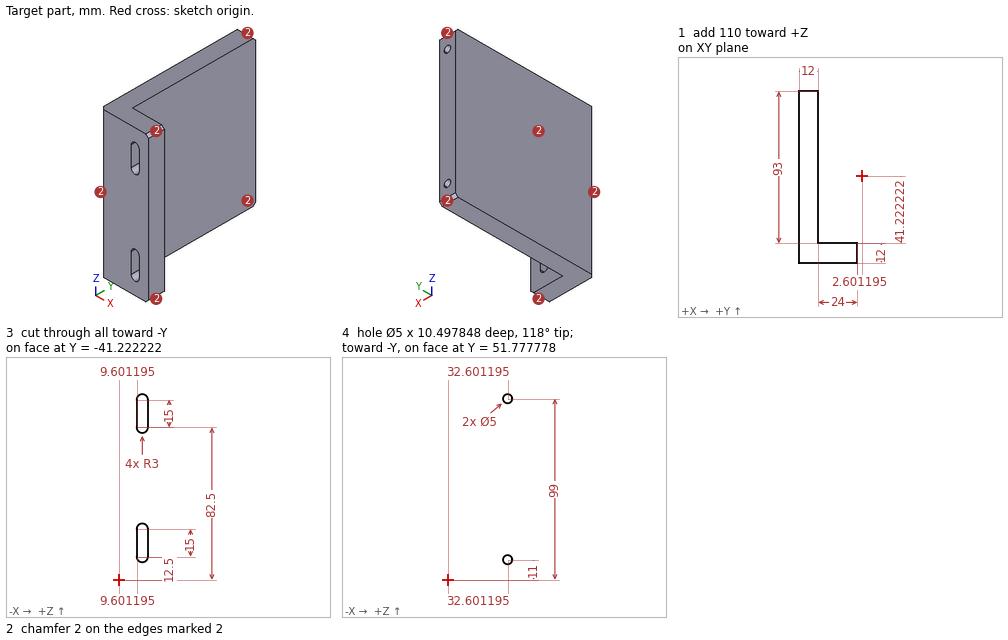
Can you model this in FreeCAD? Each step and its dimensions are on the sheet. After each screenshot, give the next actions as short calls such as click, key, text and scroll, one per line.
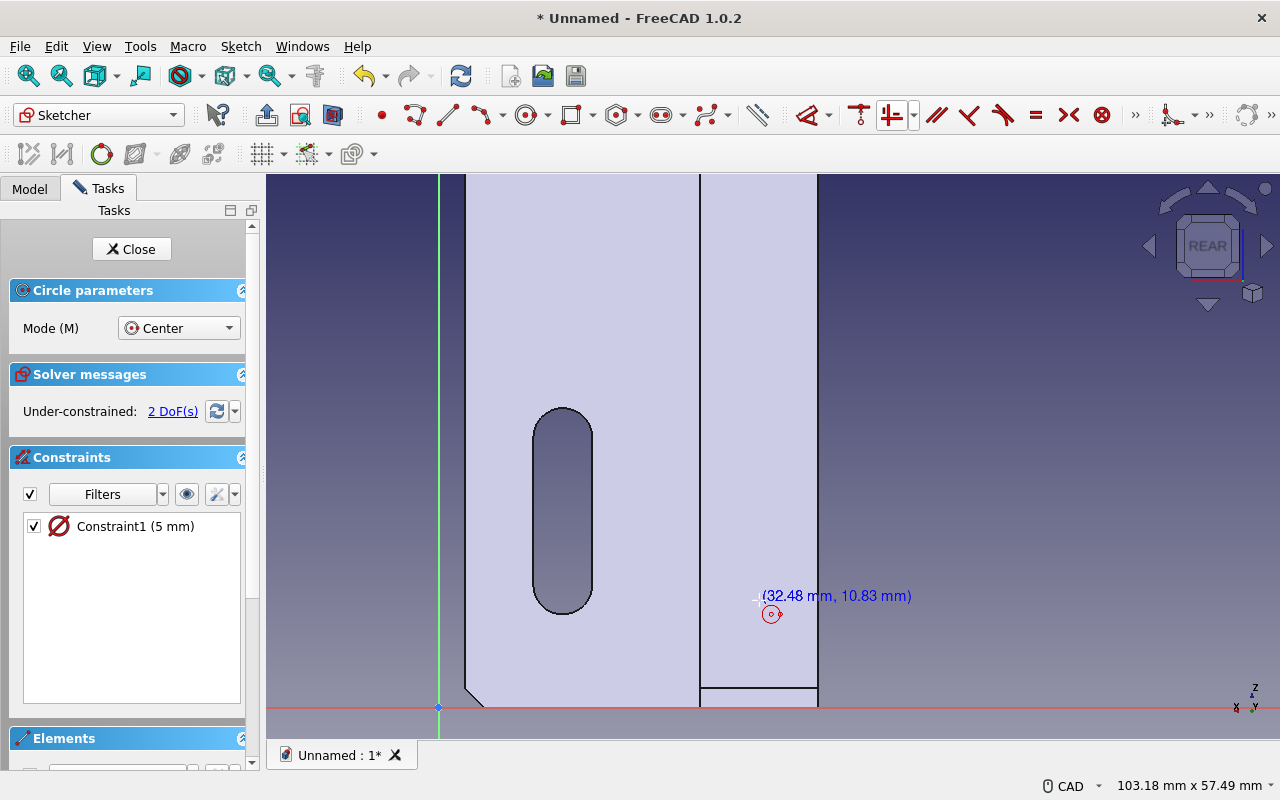
click(759, 600)
move(777, 582)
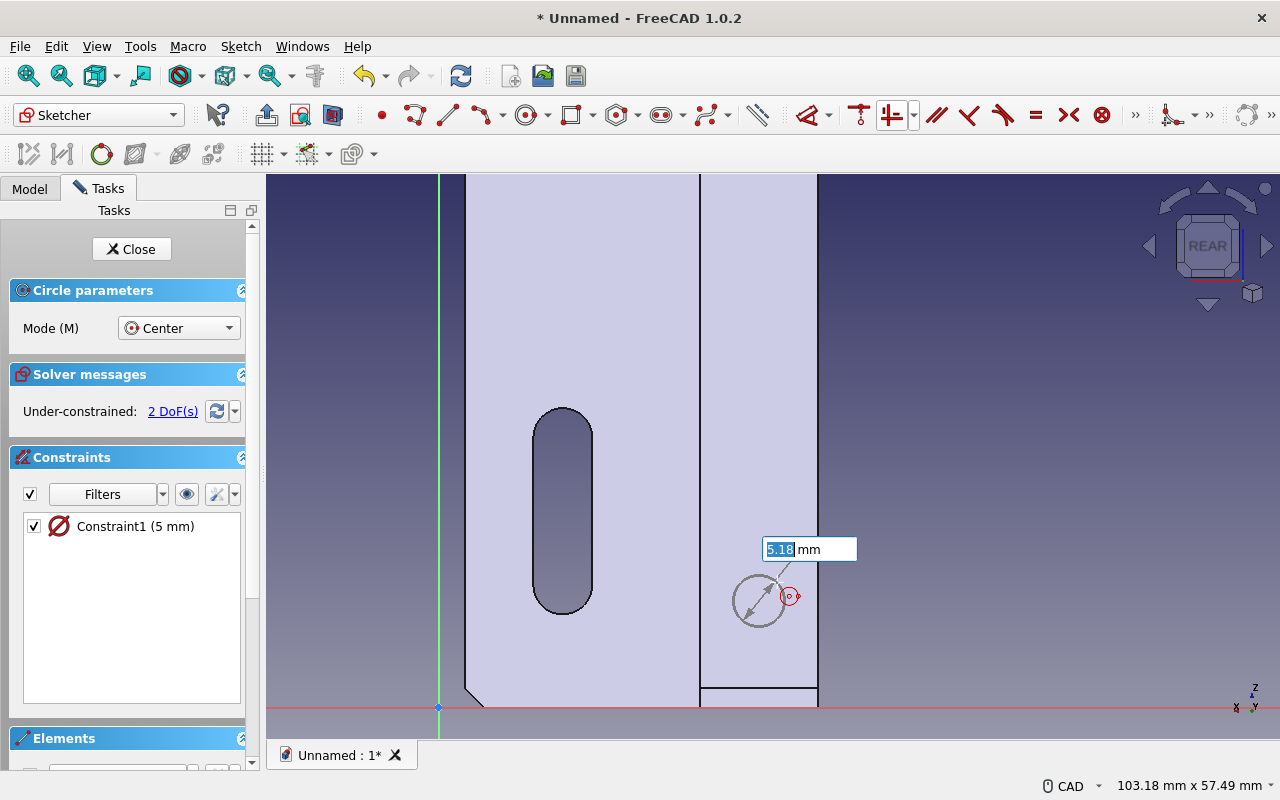
text(5)
key(Return)
key(Escape)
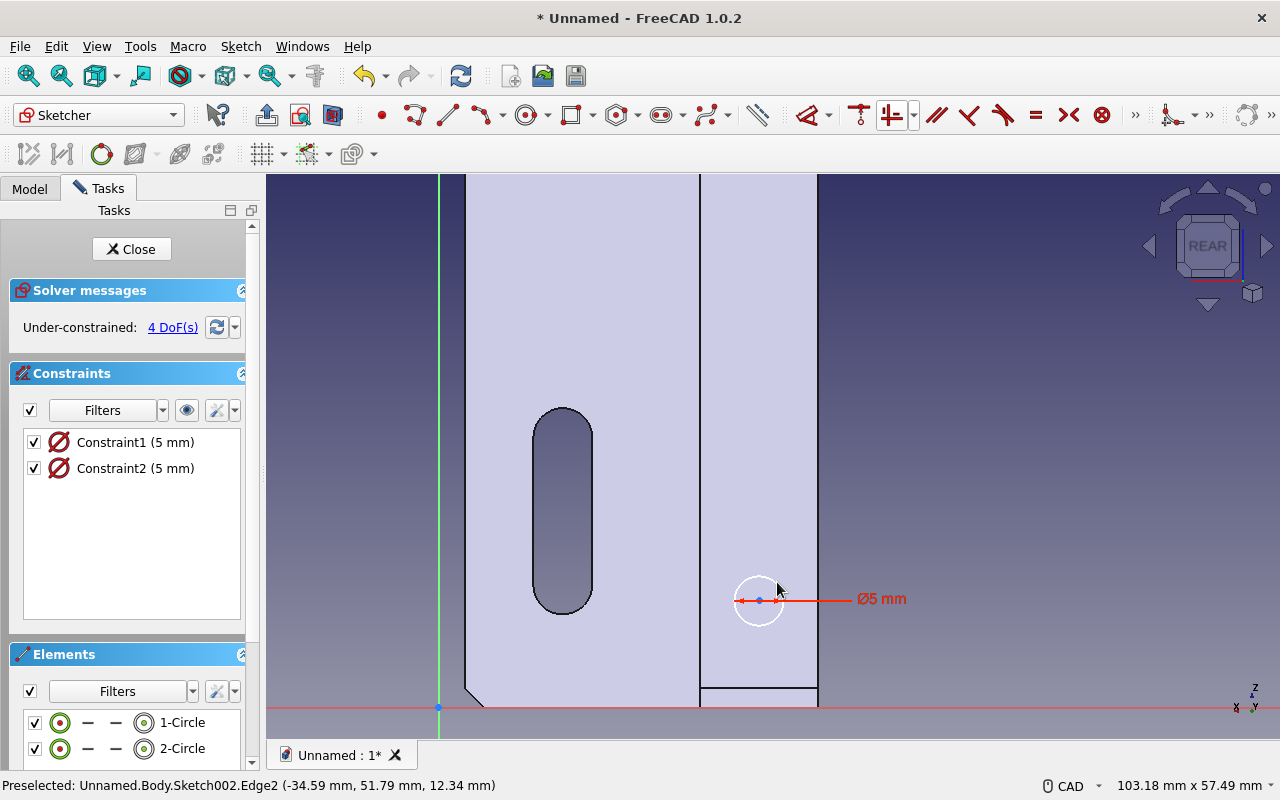
click(806, 116)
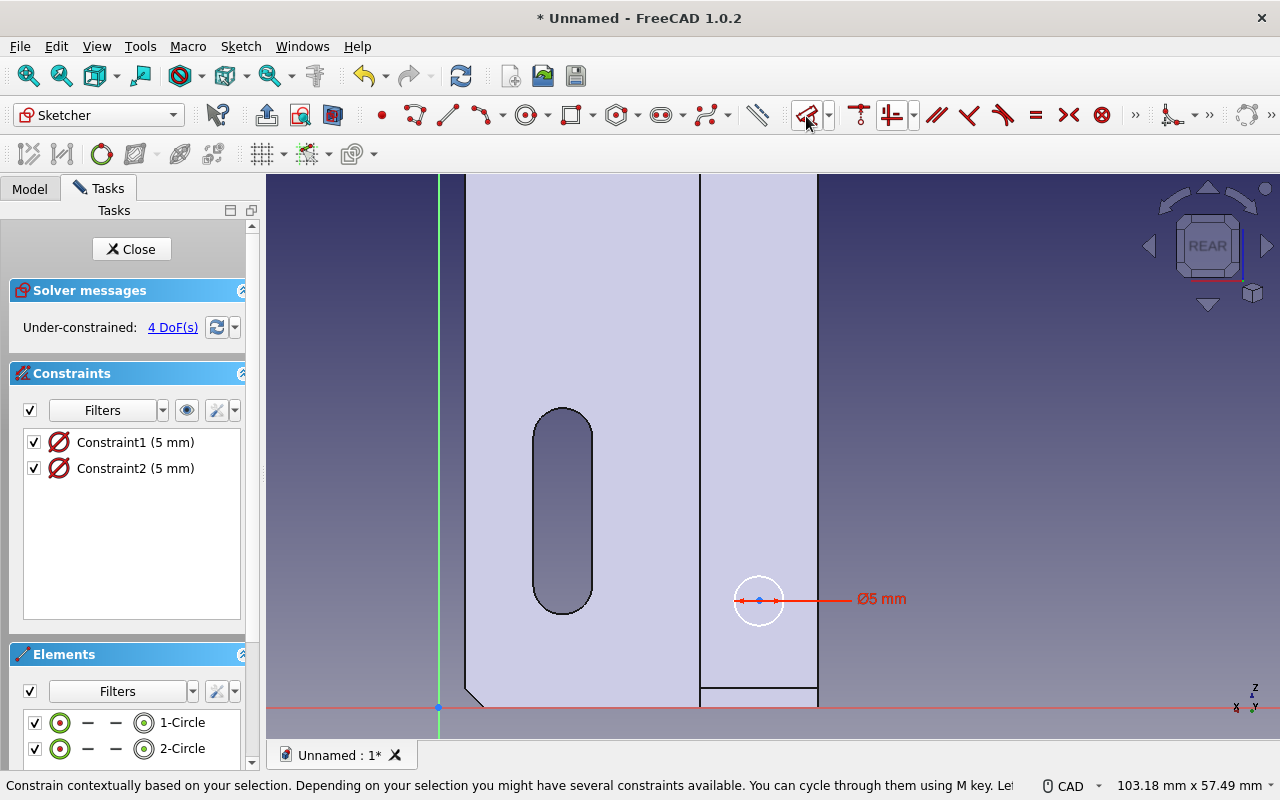
scroll(759, 600, down, 5)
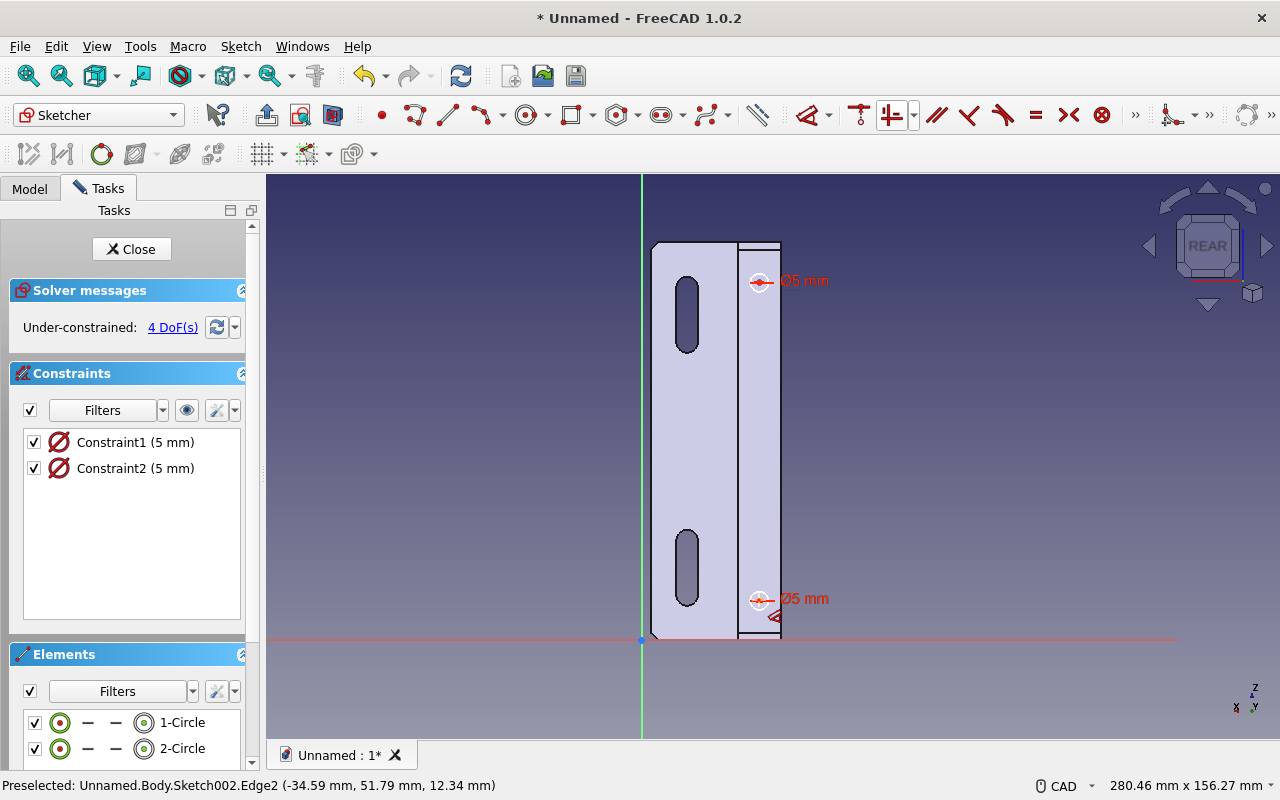
click(759, 283)
click(608, 461)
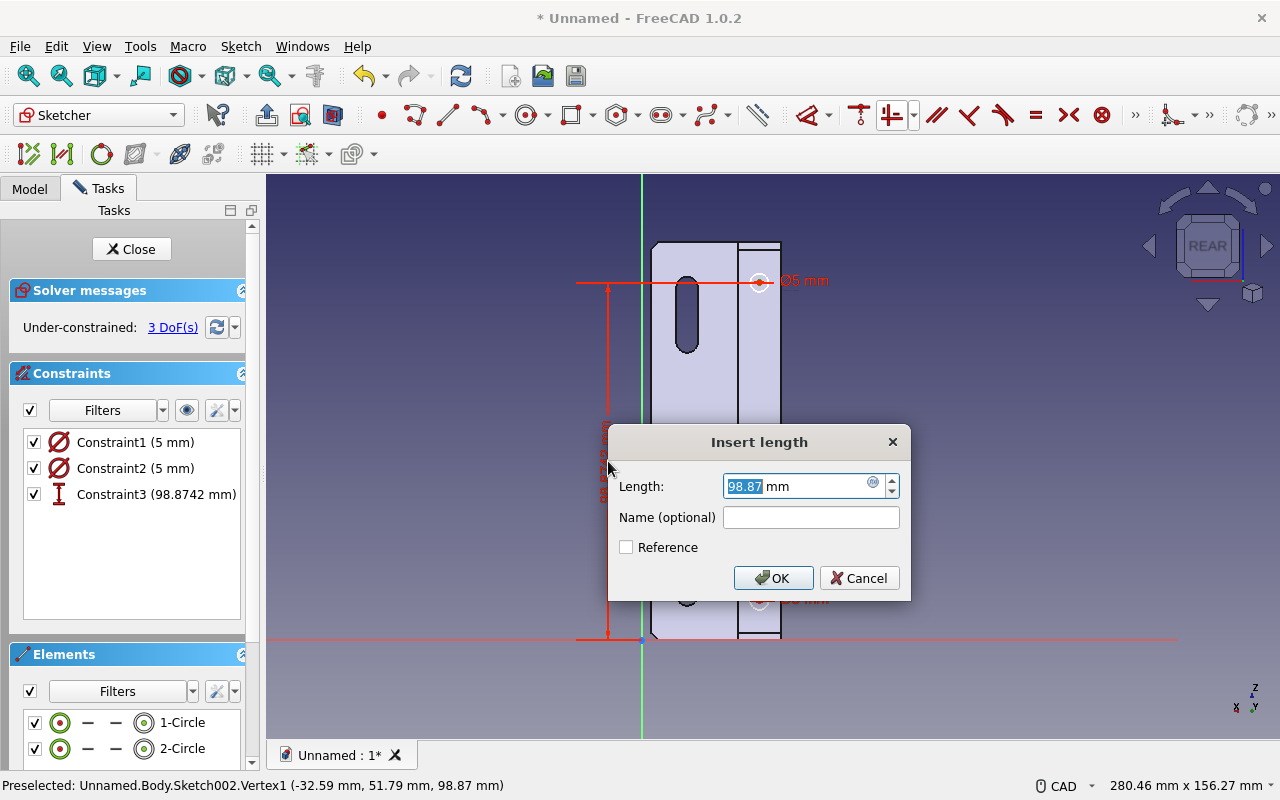
text(99)
key(Return)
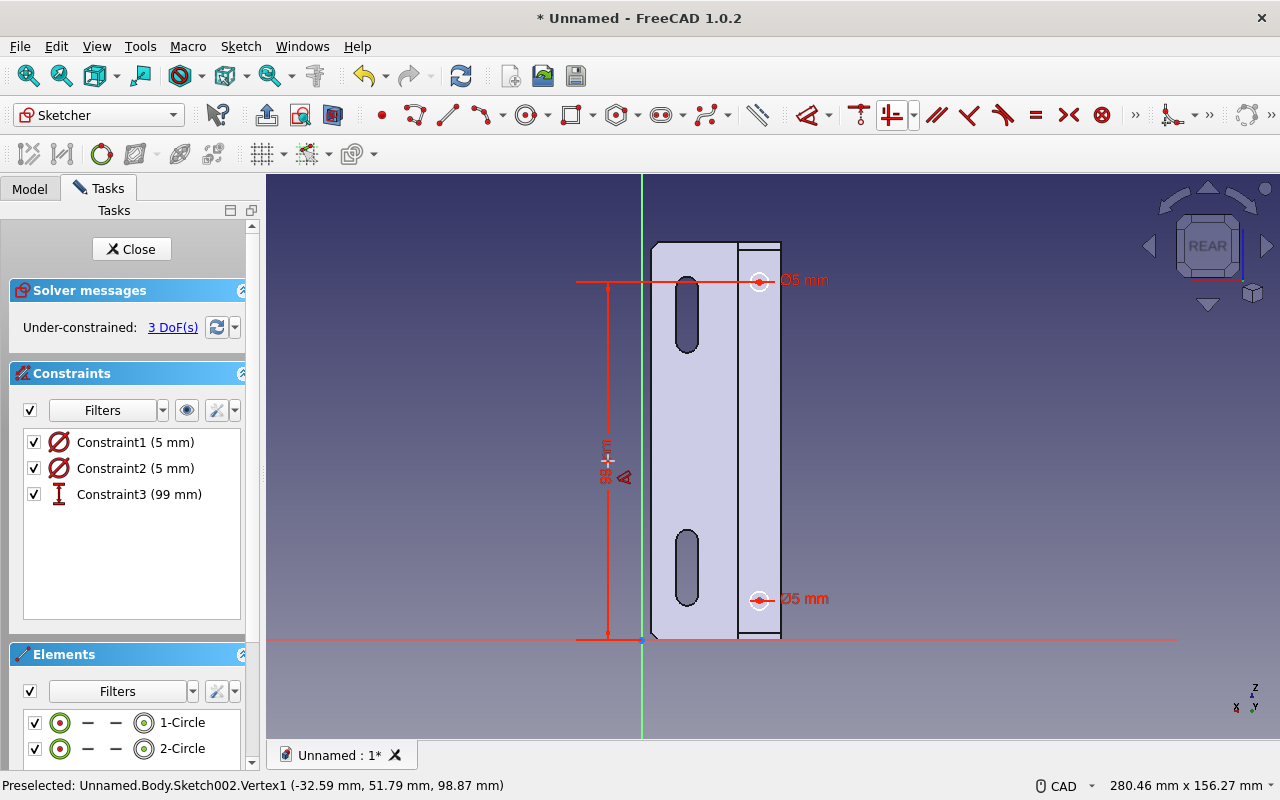
click(759, 601)
click(608, 620)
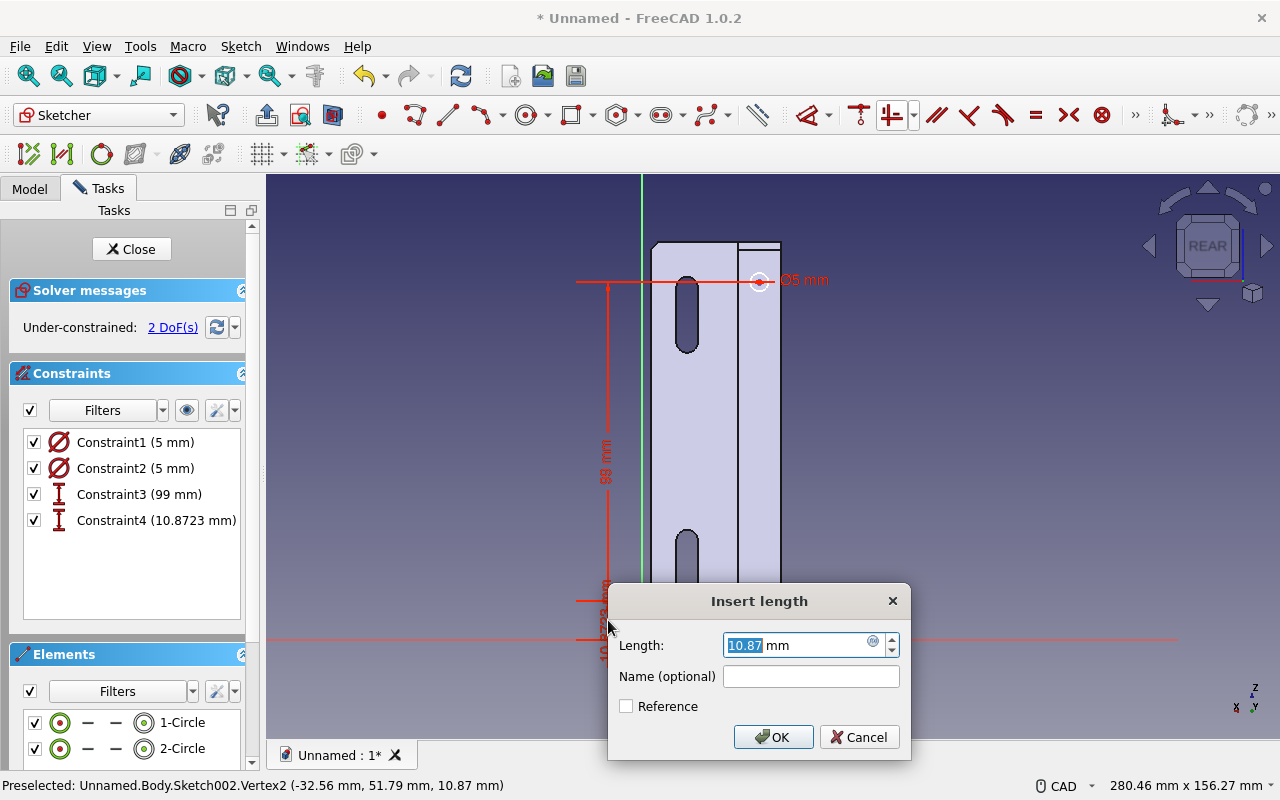
text(11)
key(Return)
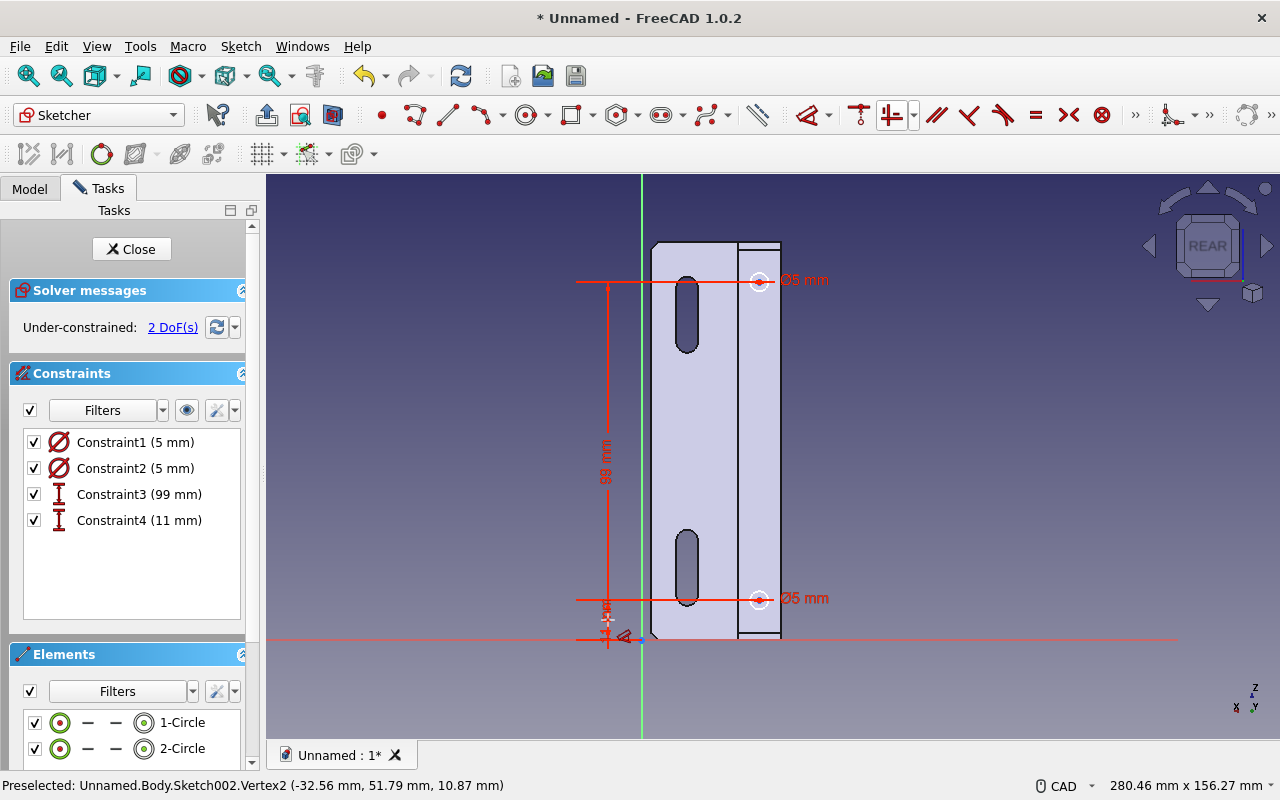
click(759, 282)
click(700, 674)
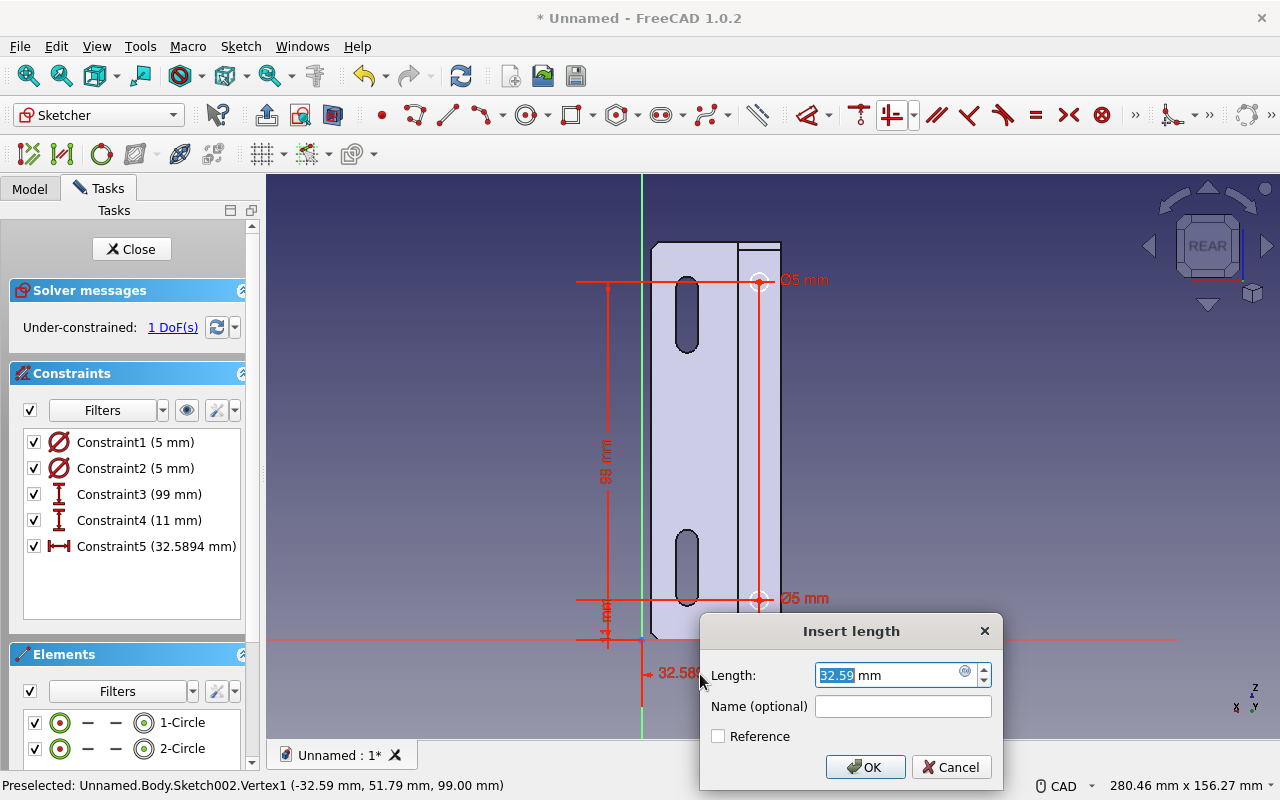
text(32.601195)
key(Return)